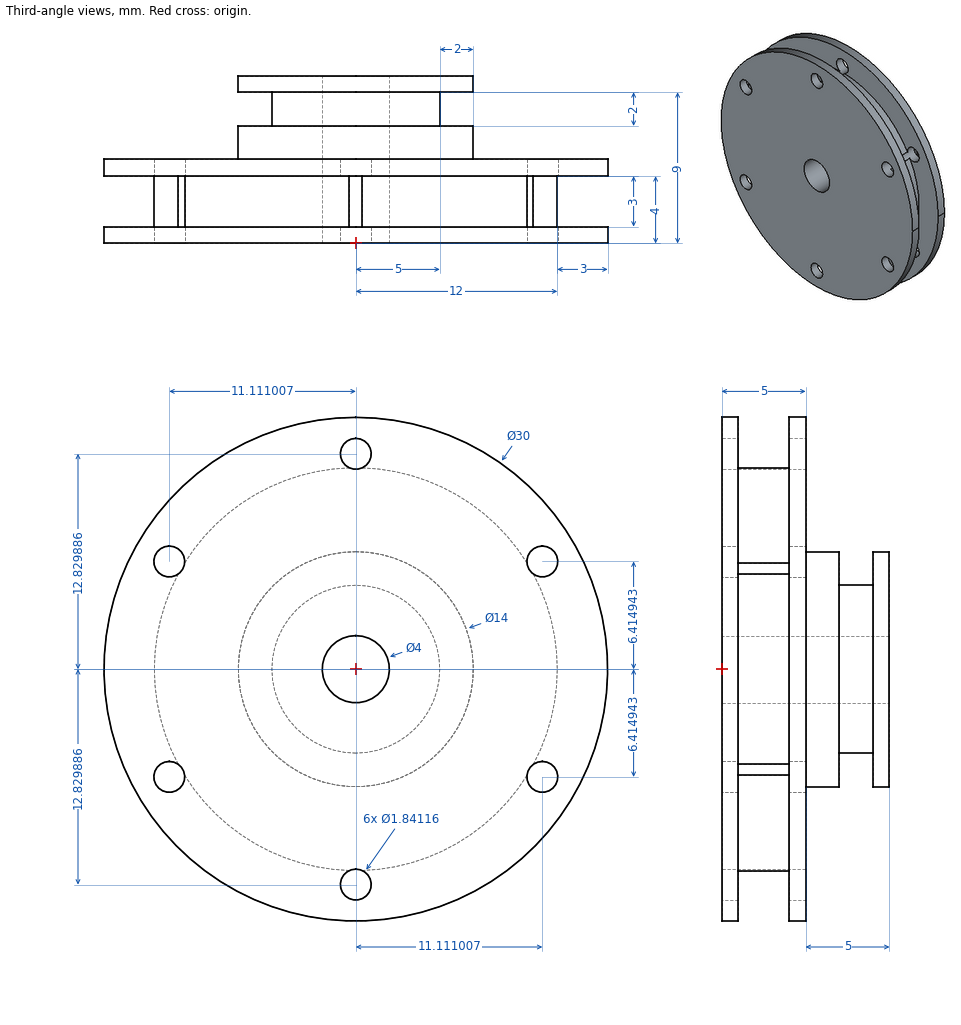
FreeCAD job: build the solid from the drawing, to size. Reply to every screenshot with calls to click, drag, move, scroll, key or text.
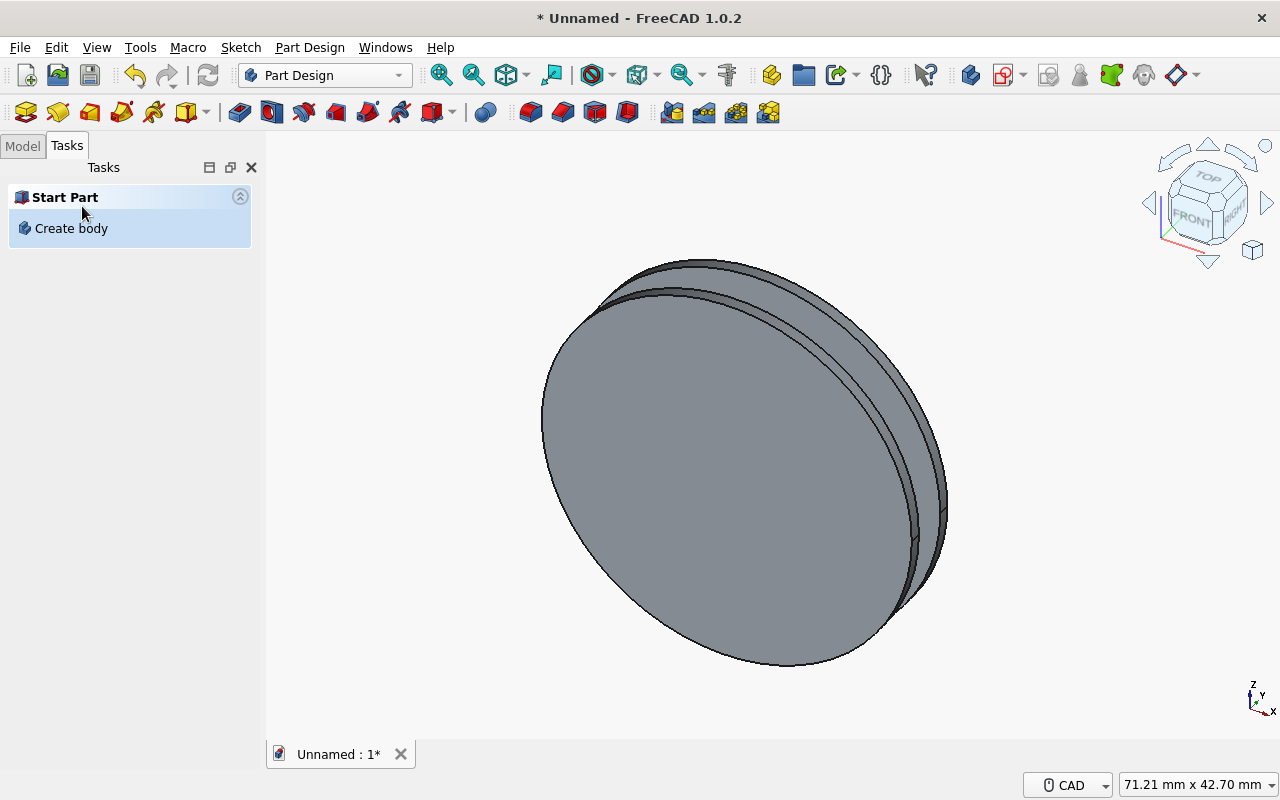
key(4)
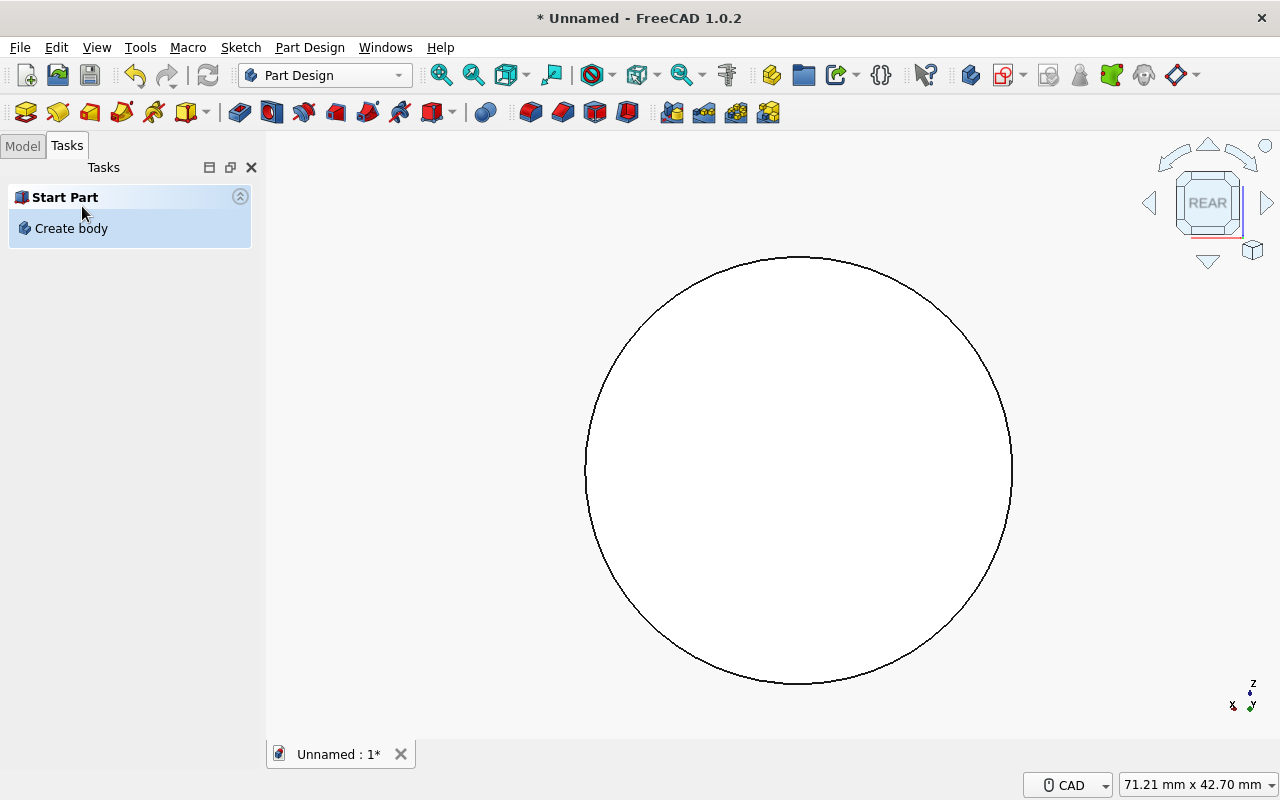
click(799, 470)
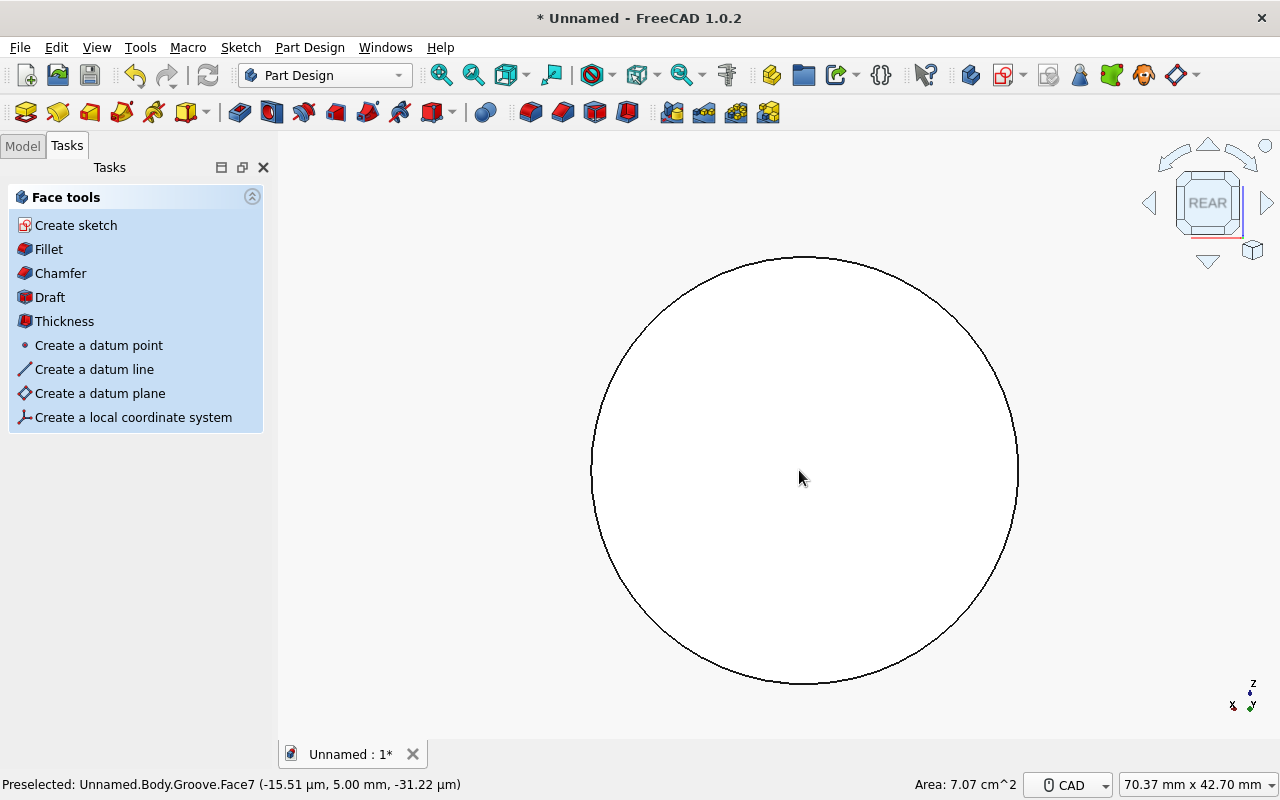
click(1004, 76)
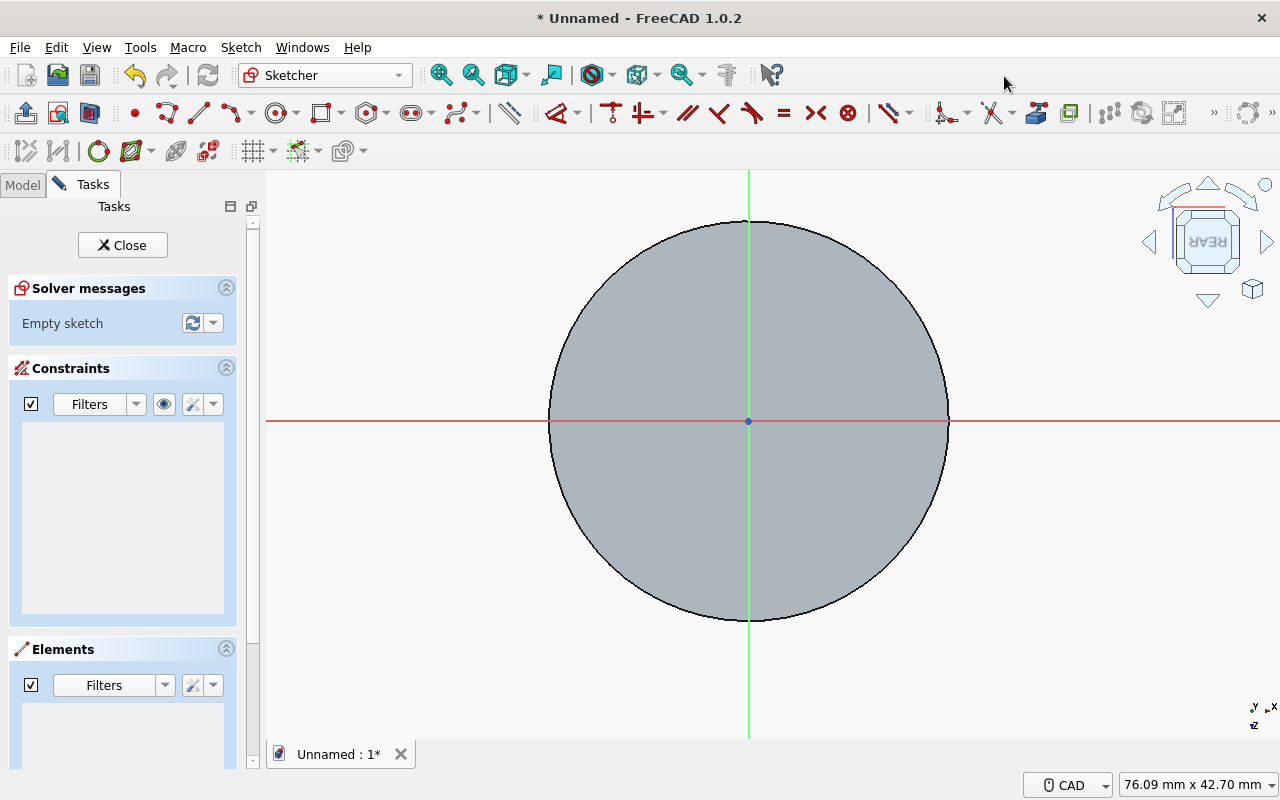
scroll(803, 381, up, 3)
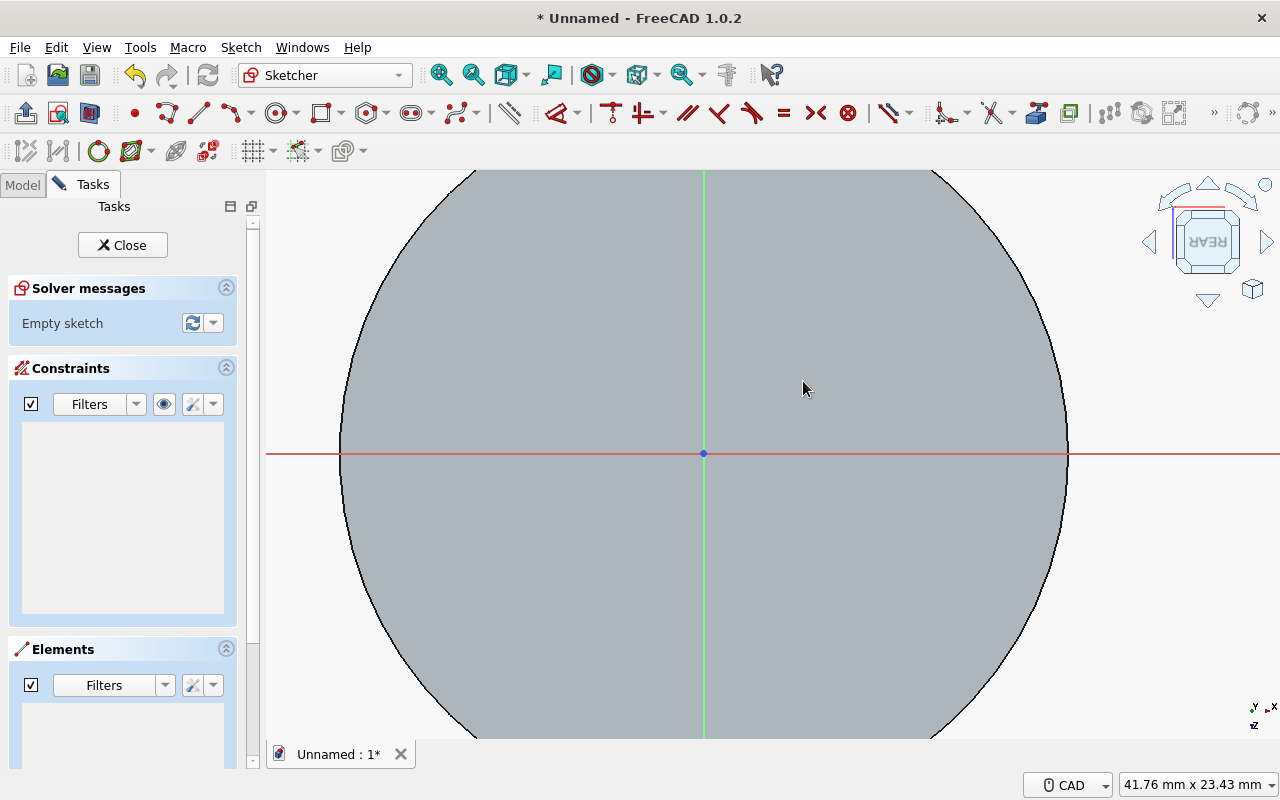
click(276, 114)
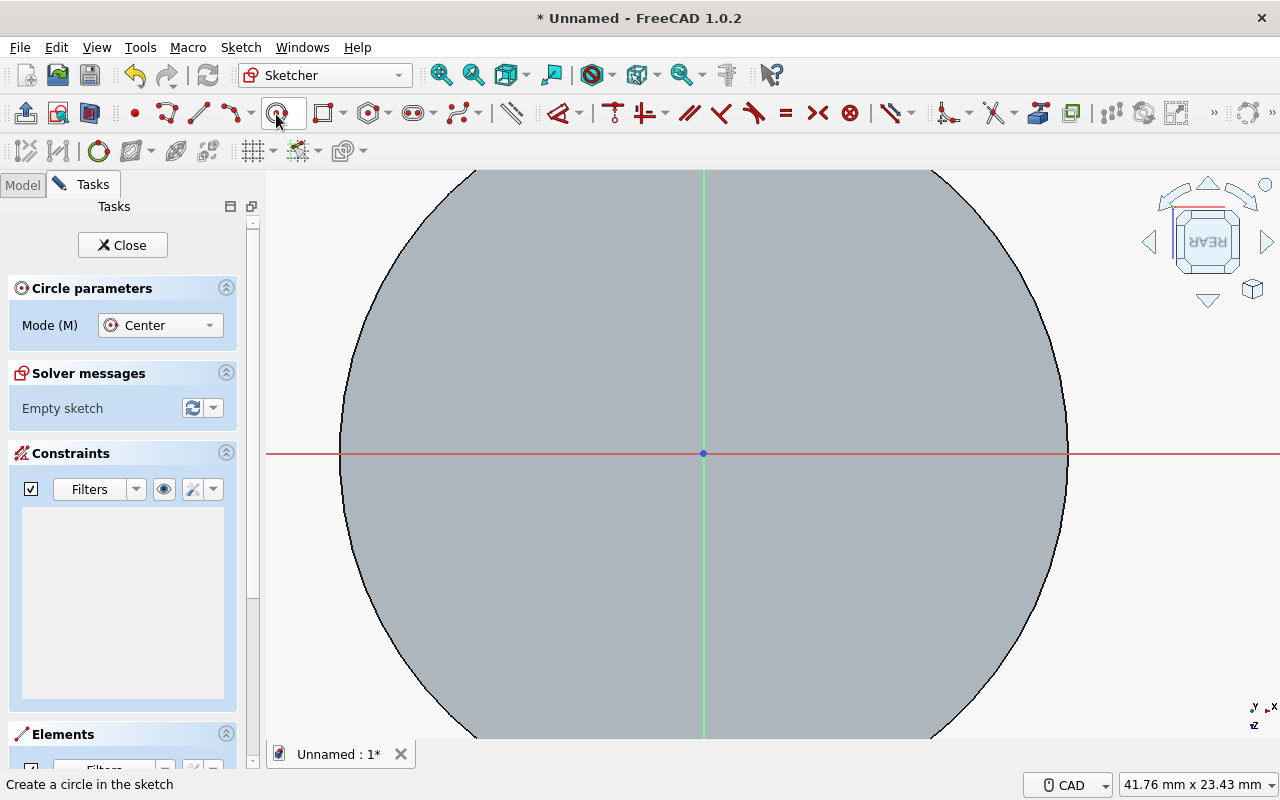
click(704, 454)
move(824, 334)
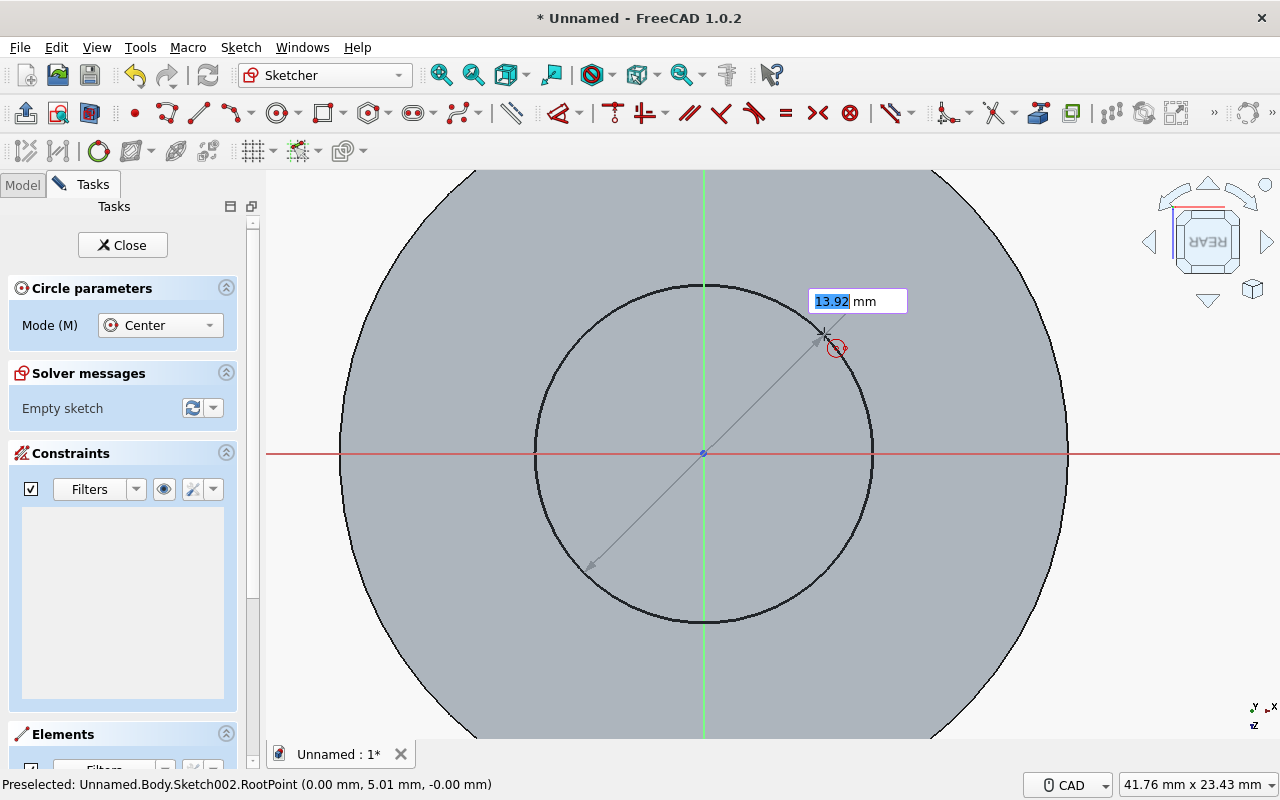
text(14)
key(Return)
key(Escape)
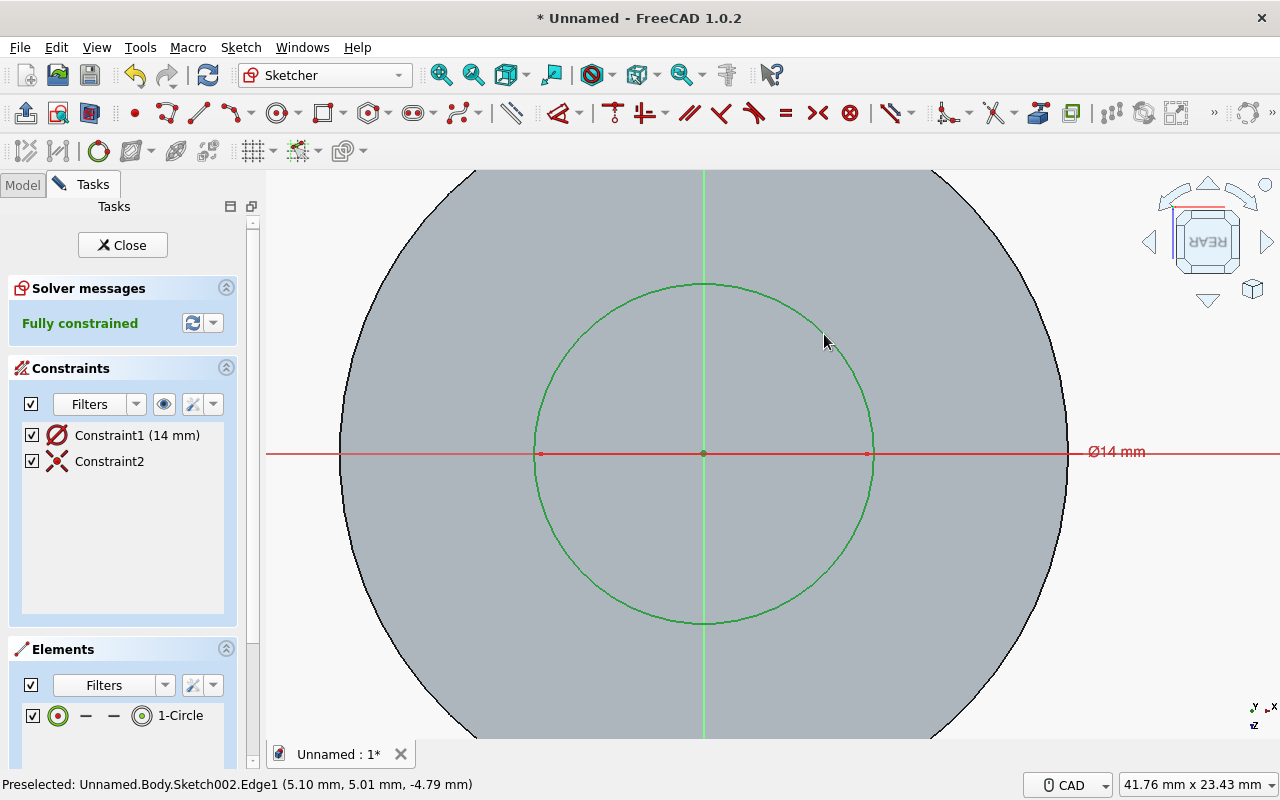
click(123, 245)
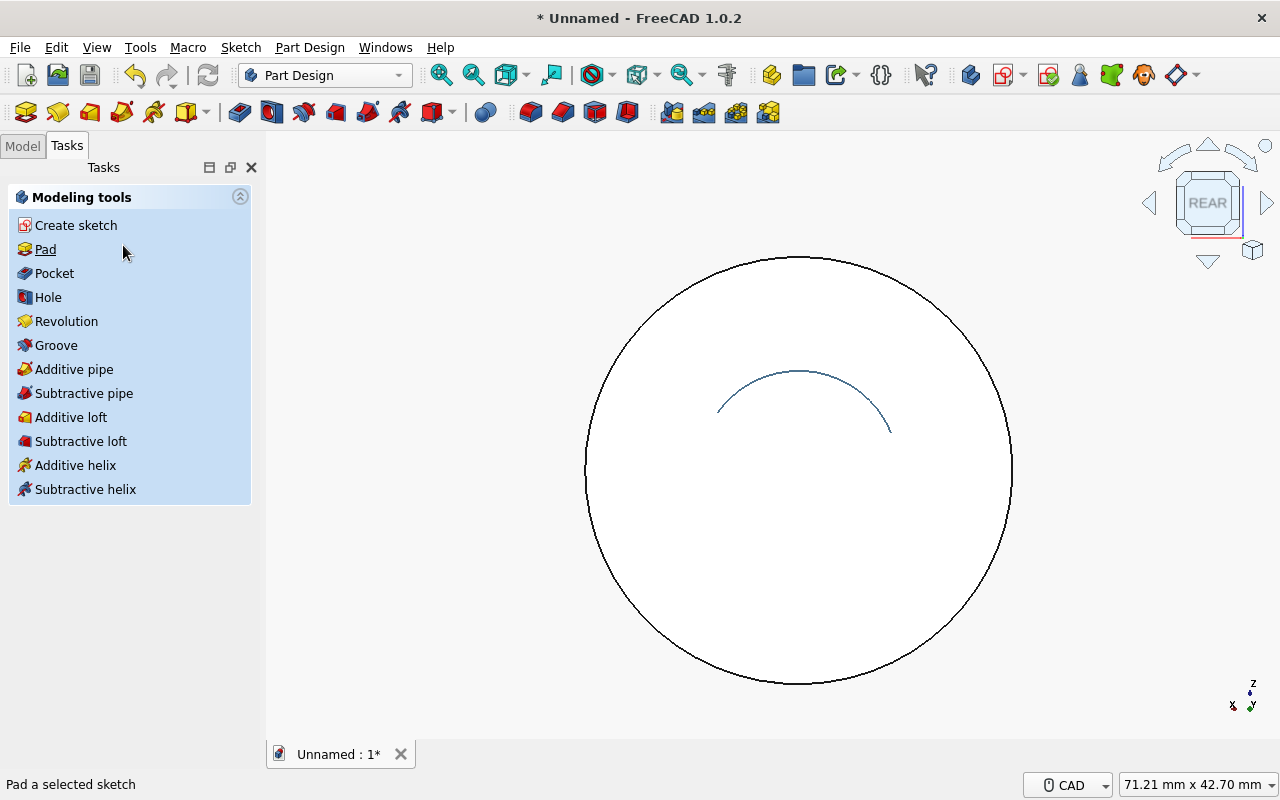
click(26, 112)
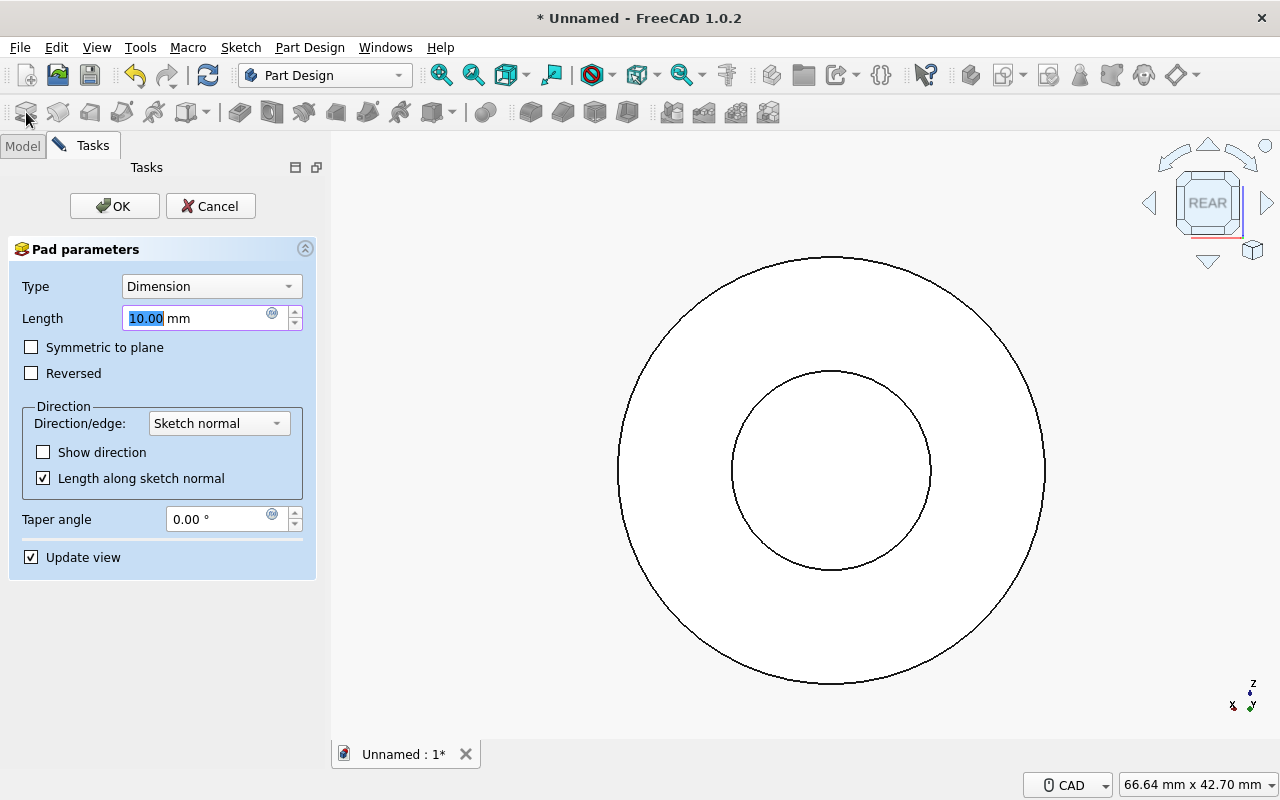
text(5)
key(Tab)